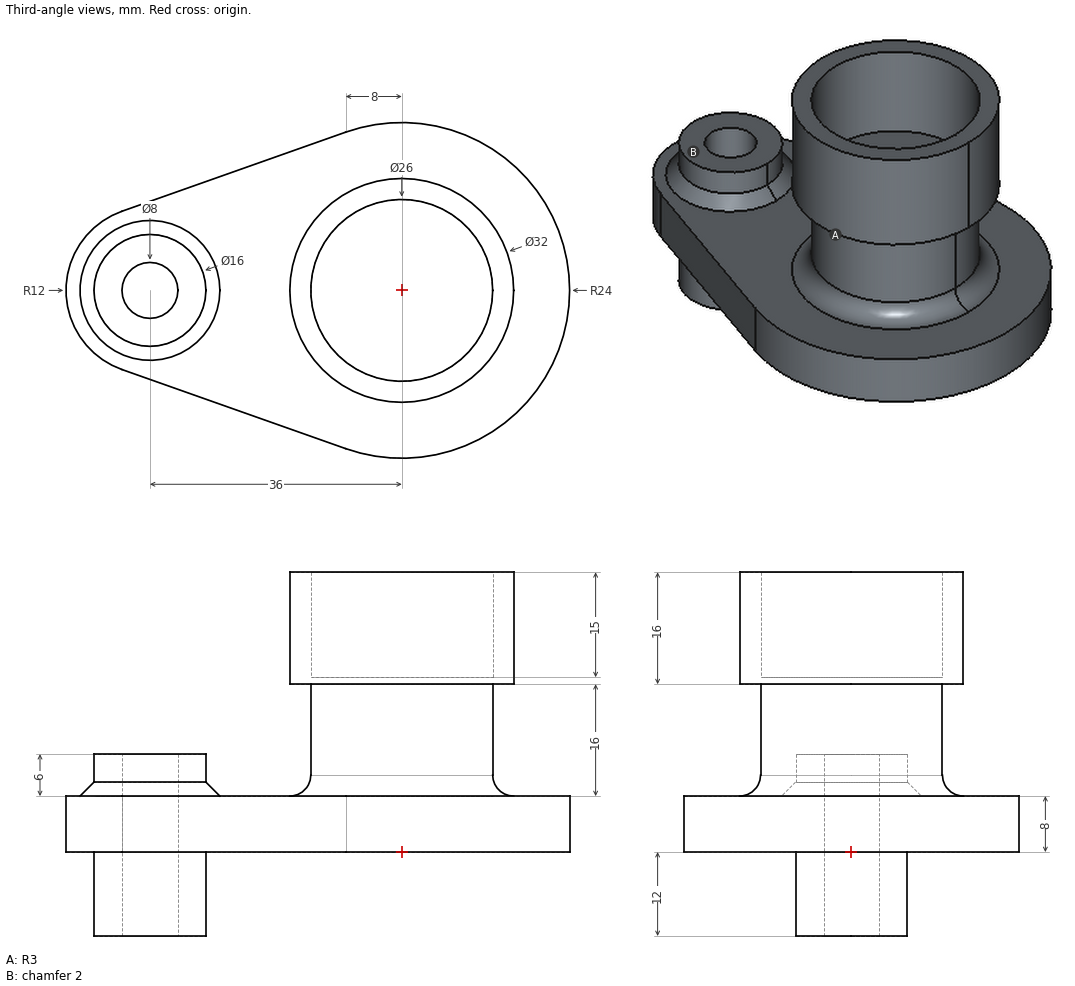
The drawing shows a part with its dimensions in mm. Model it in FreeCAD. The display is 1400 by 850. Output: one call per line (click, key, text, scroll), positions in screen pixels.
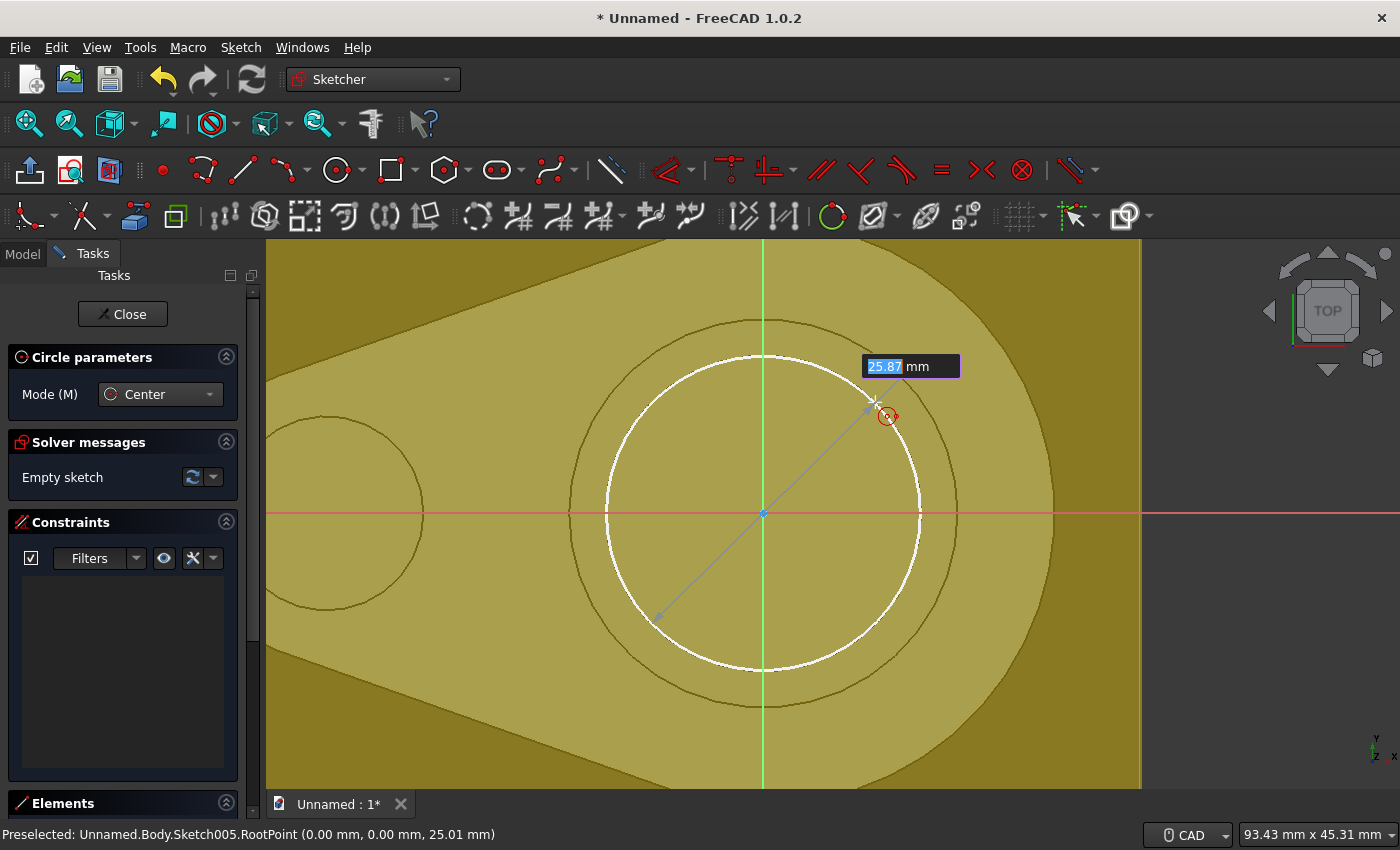
text(26)
key(Return)
key(Escape)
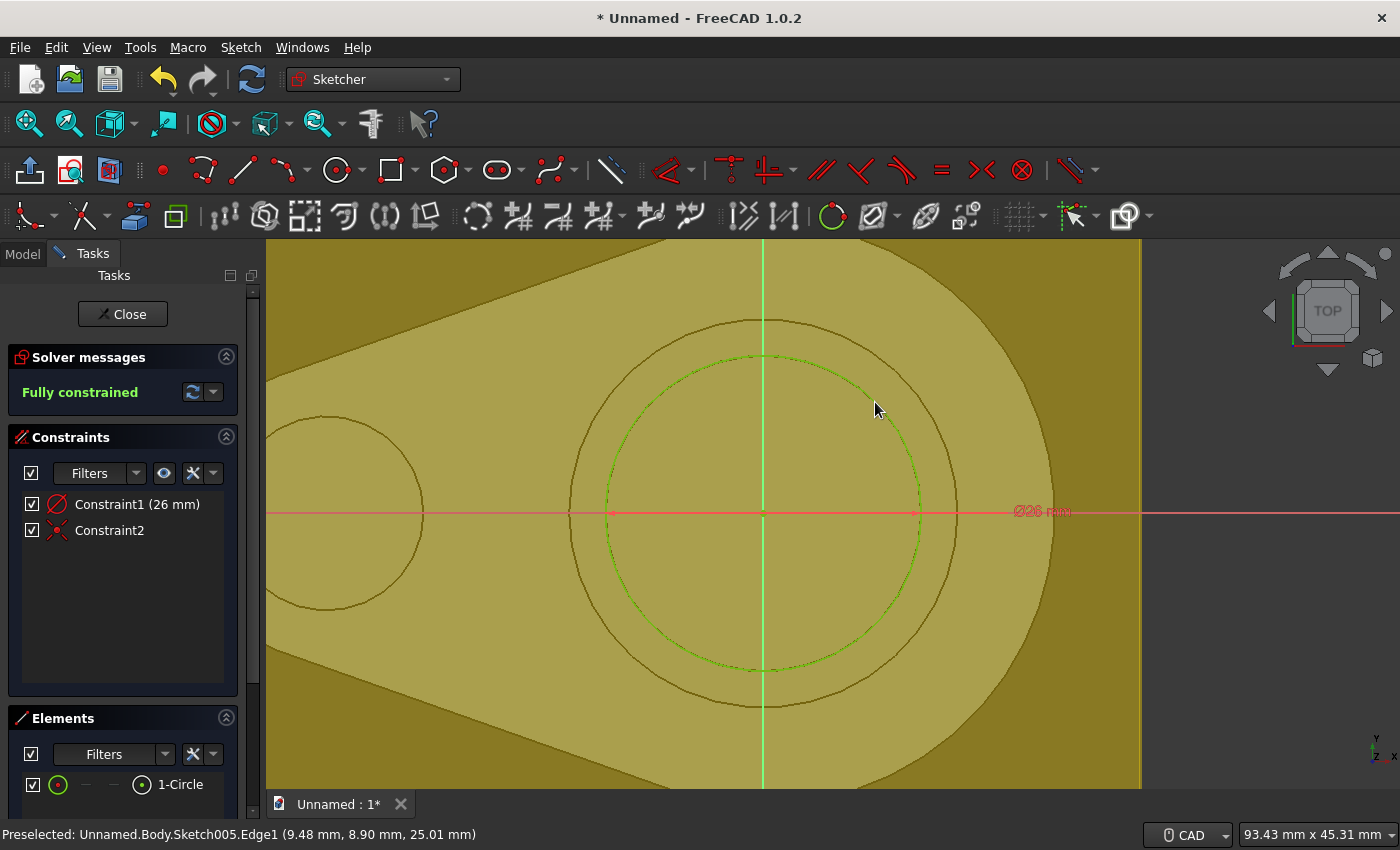
click(123, 314)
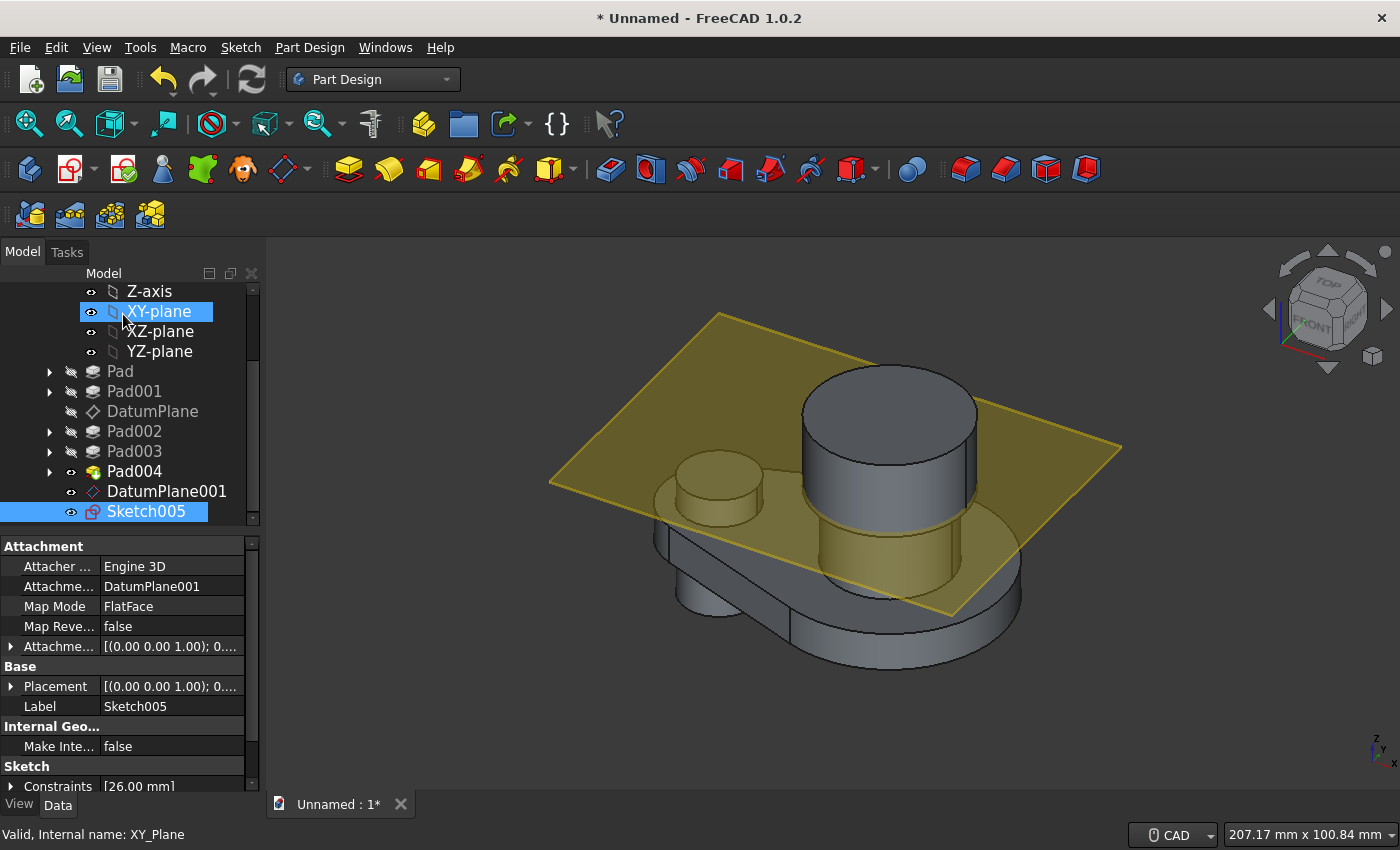
click(612, 170)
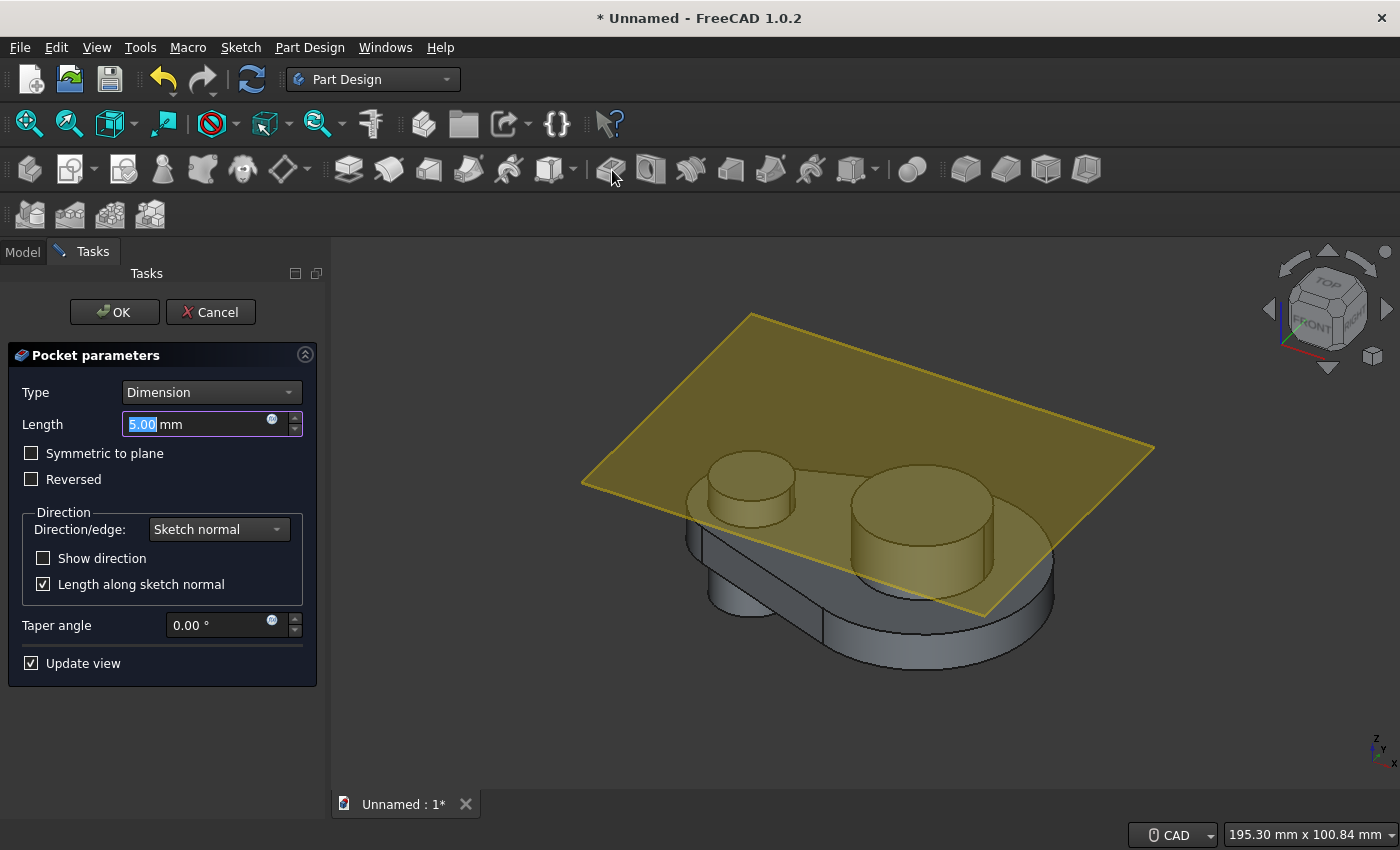
text(15)
key(Tab)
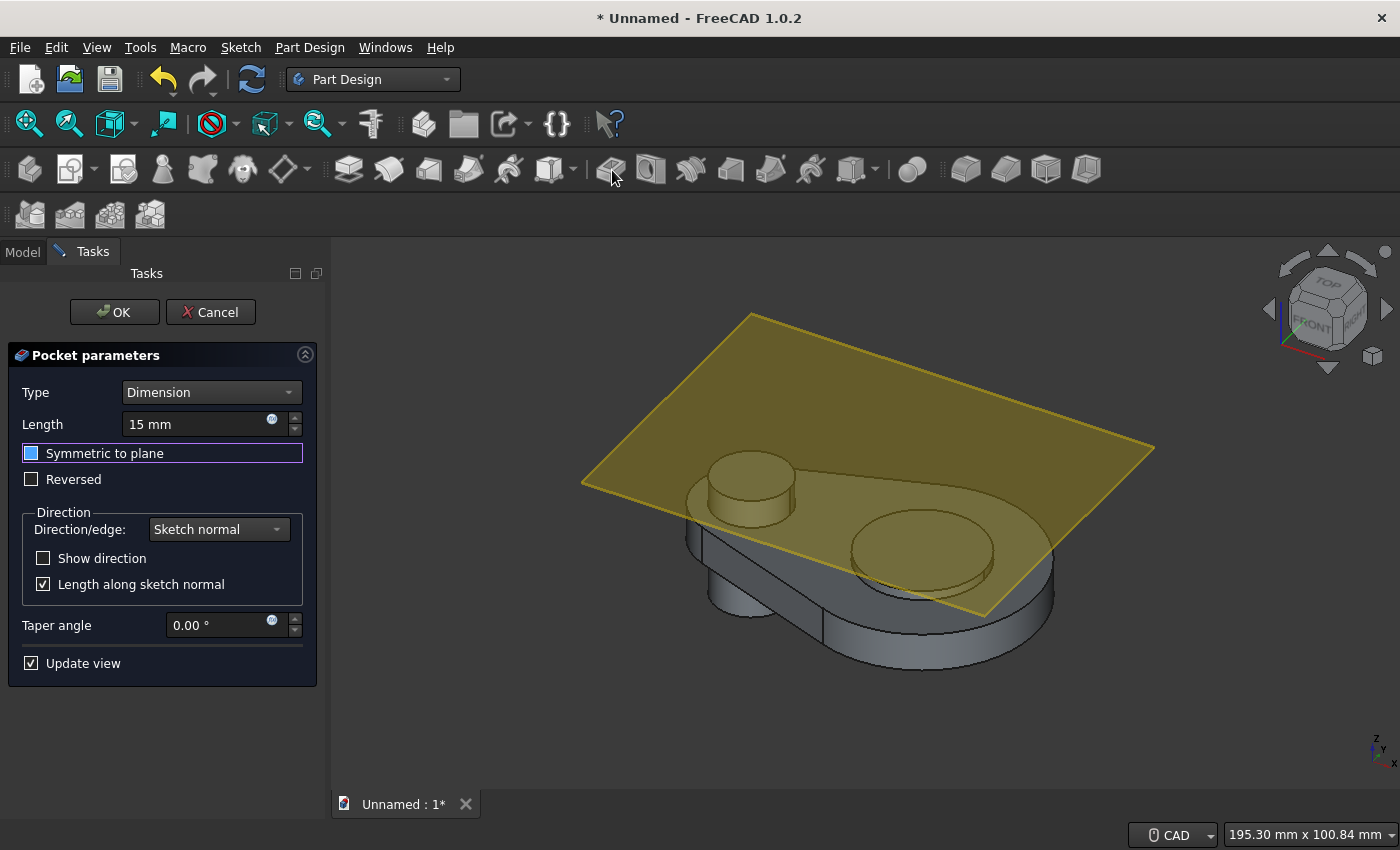
click(30, 479)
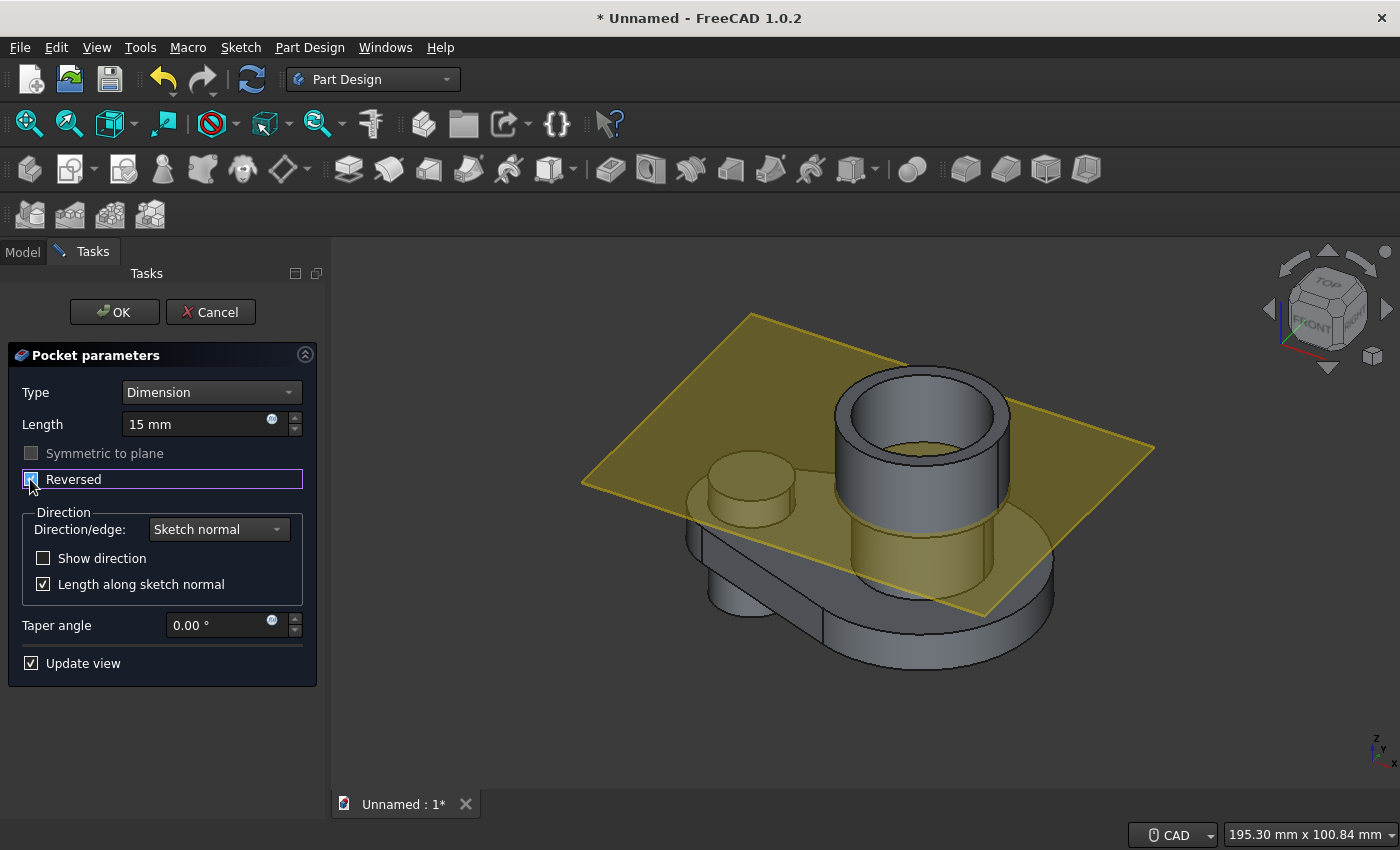
click(115, 312)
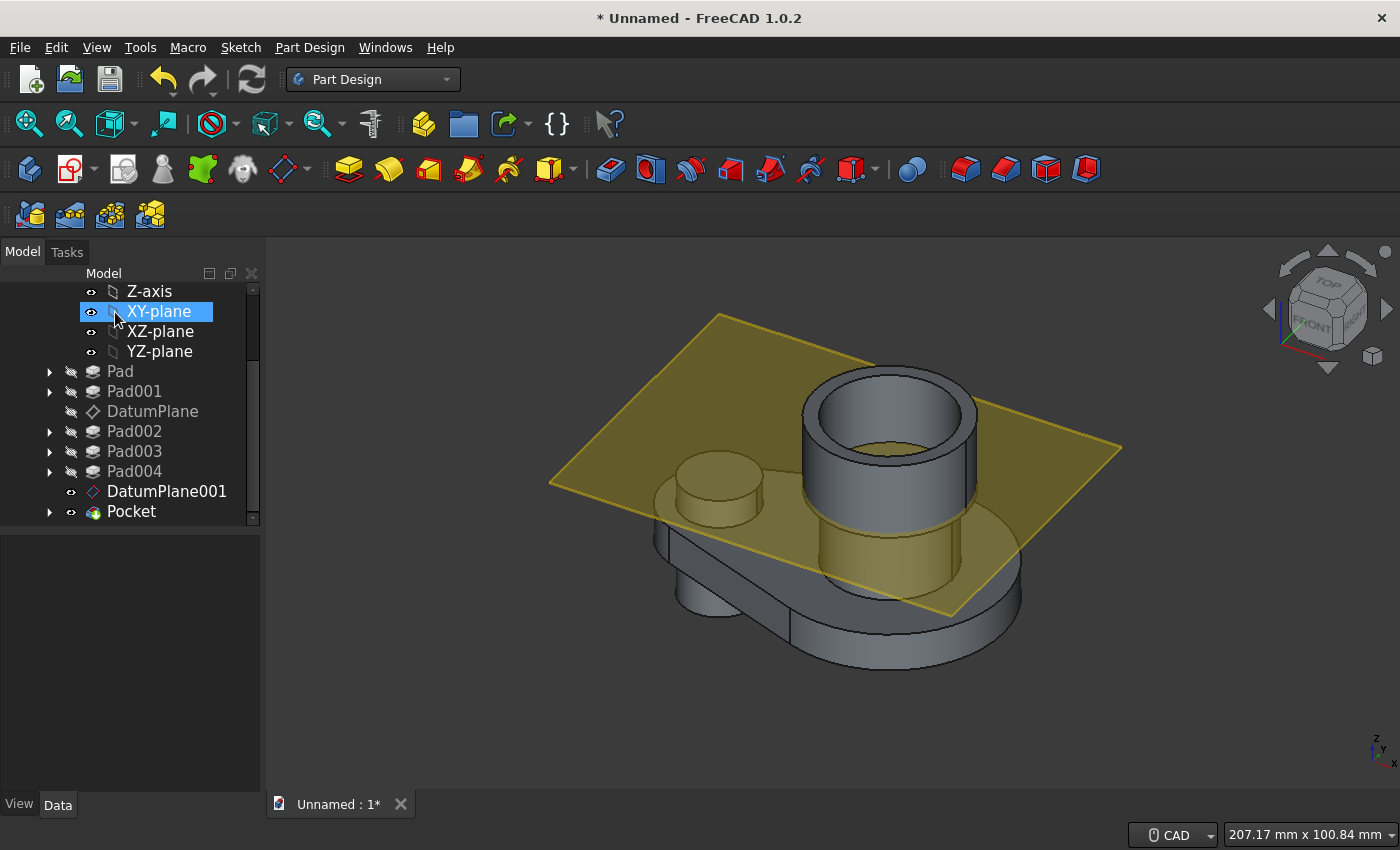
click(116, 492)
key(space)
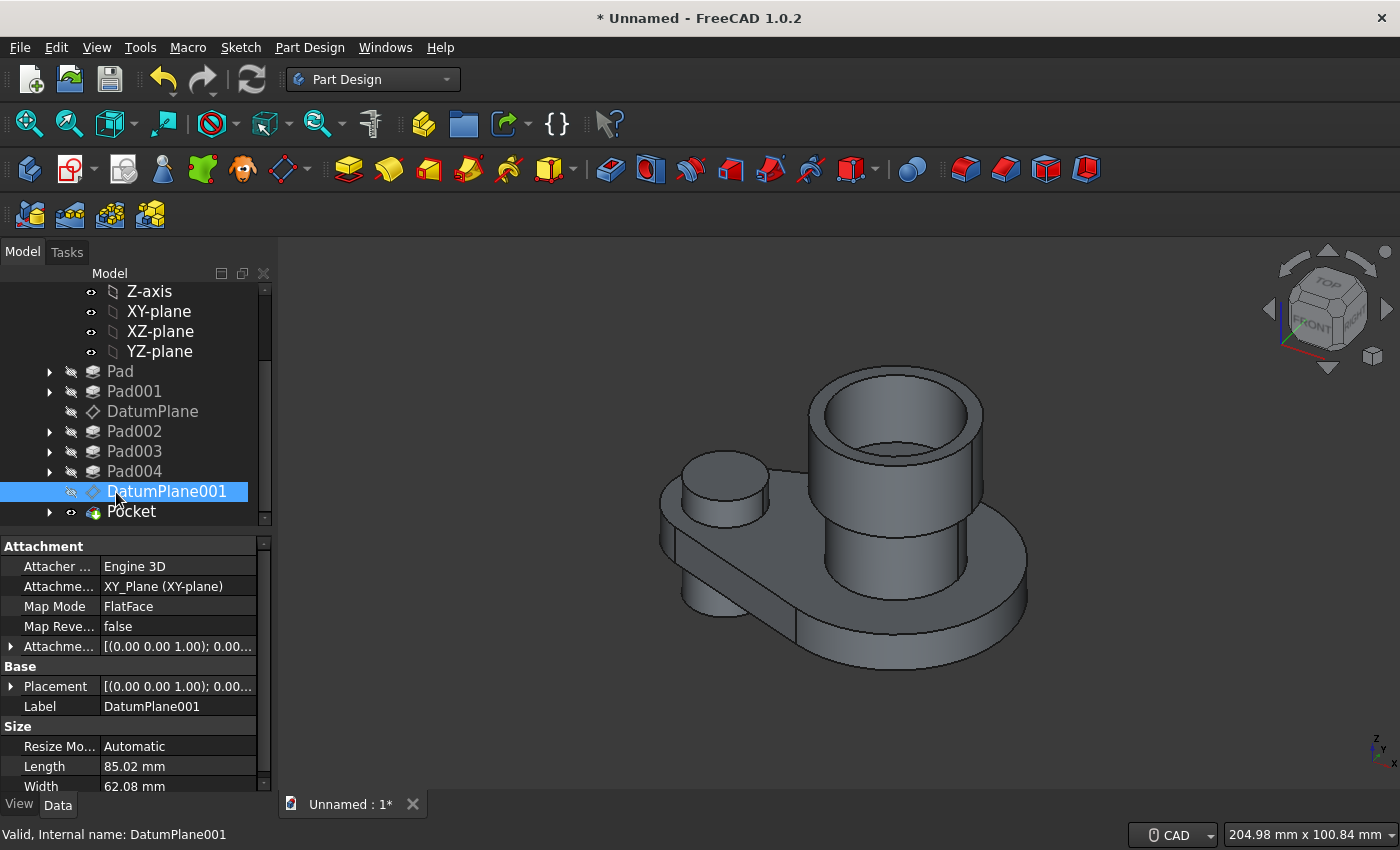
key(0)